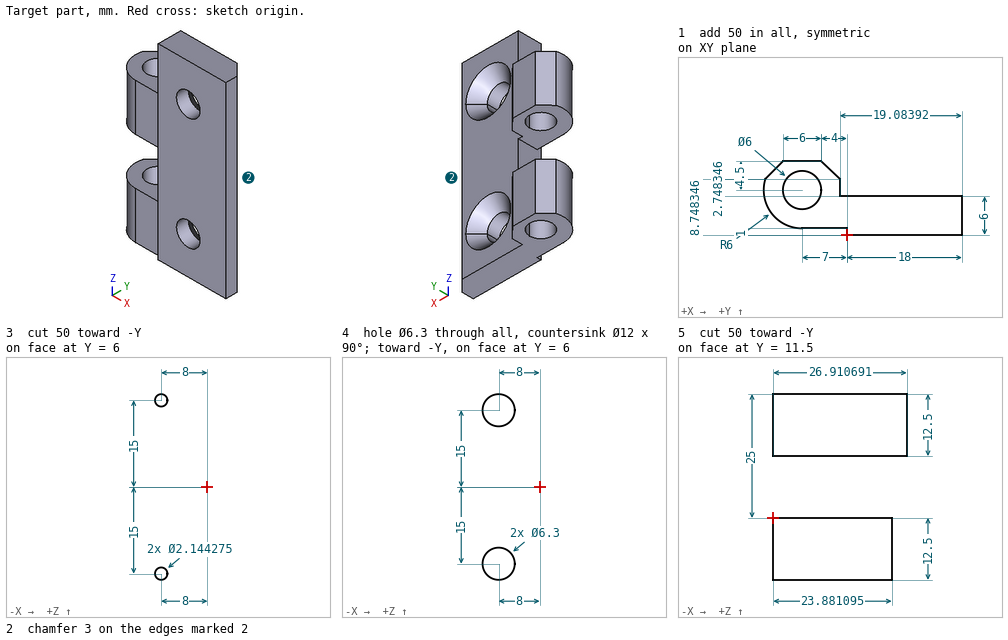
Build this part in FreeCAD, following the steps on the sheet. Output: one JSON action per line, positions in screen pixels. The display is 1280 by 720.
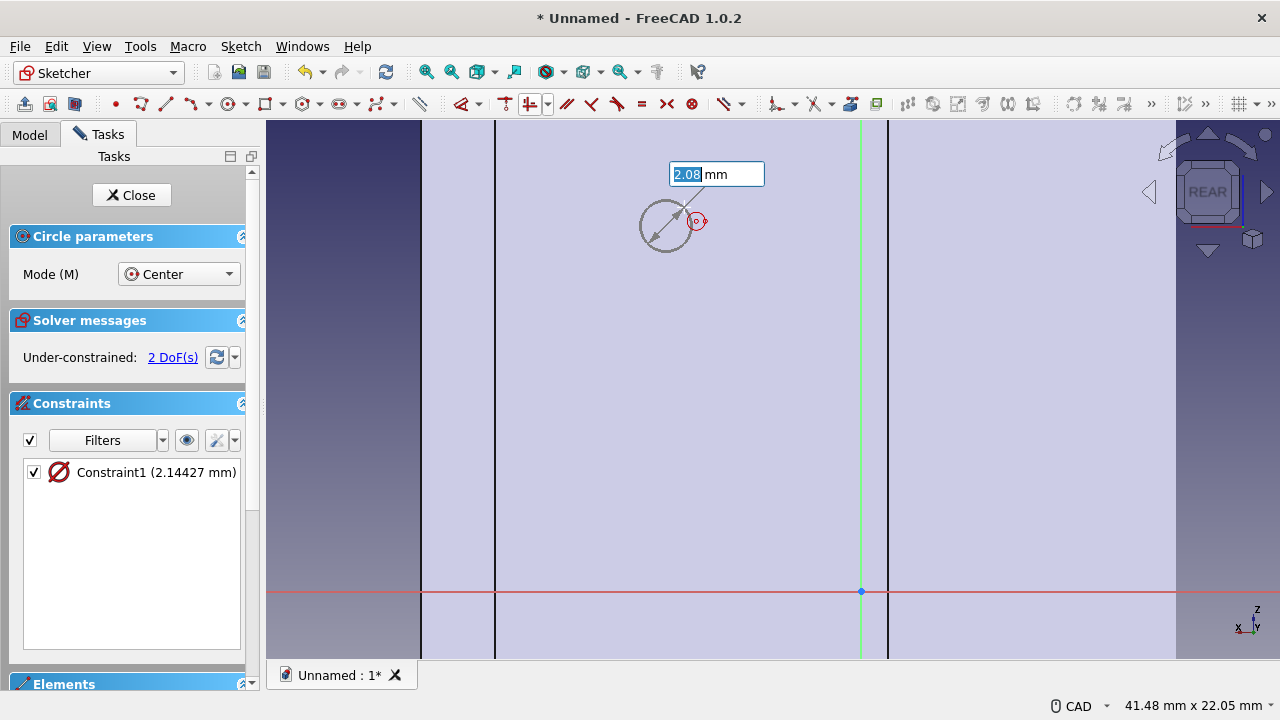
{"action": "type", "text": "2.144275"}
{"action": "key", "text": "Return"}
{"action": "key", "text": "Escape"}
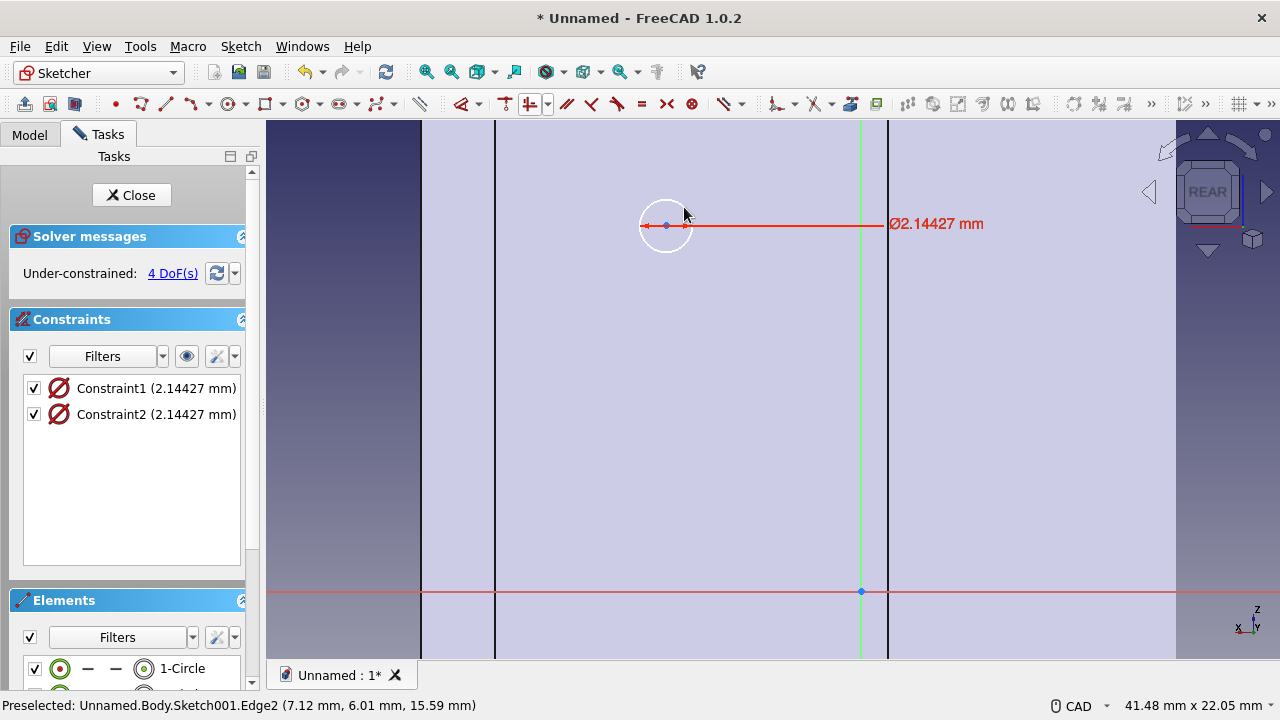
{"action": "left_click", "coordinate": [460, 104]}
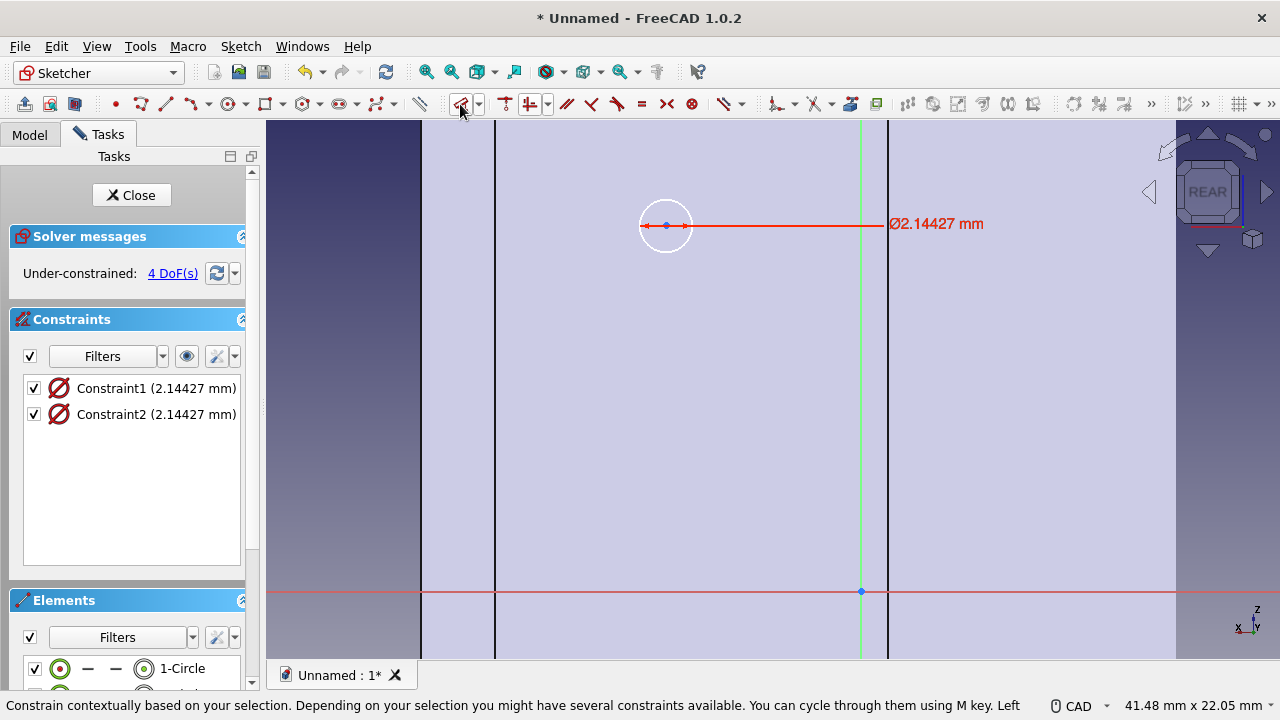
{"action": "scroll", "coordinate": [667, 224], "scroll_direction": "down", "scroll_amount": 4}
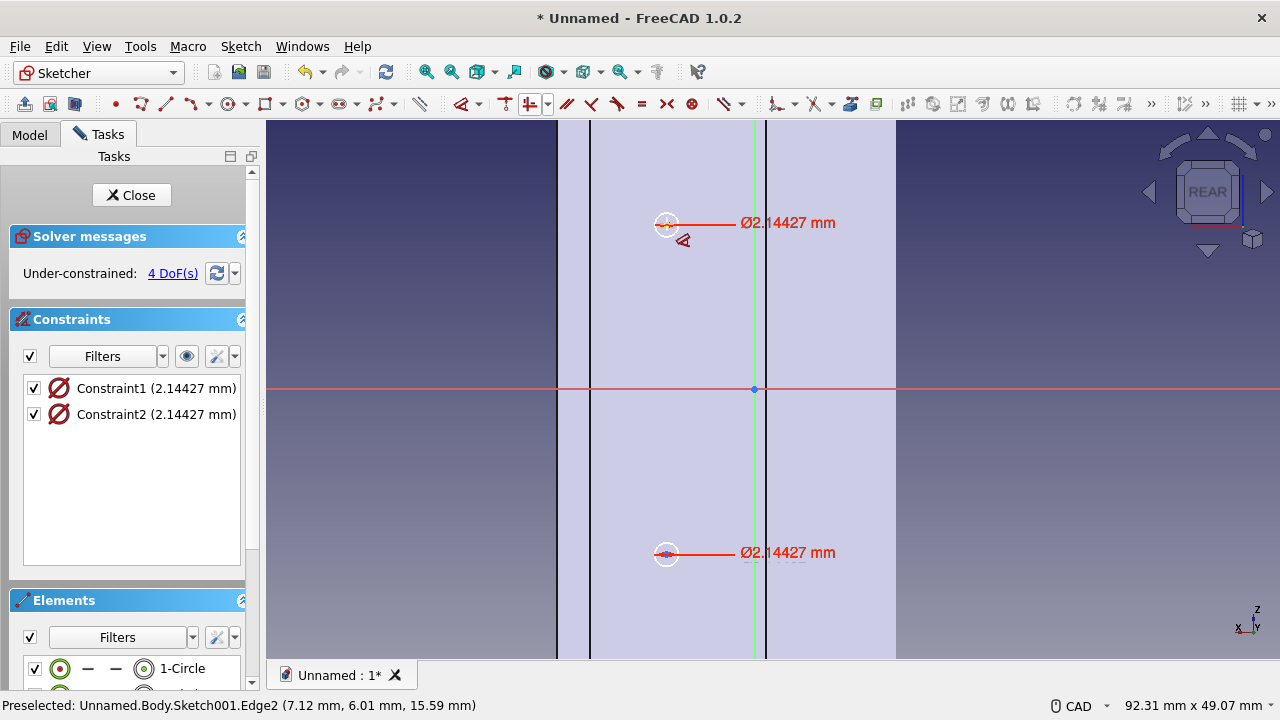
{"action": "left_click", "coordinate": [667, 555]}
{"action": "left_click", "coordinate": [711, 589]}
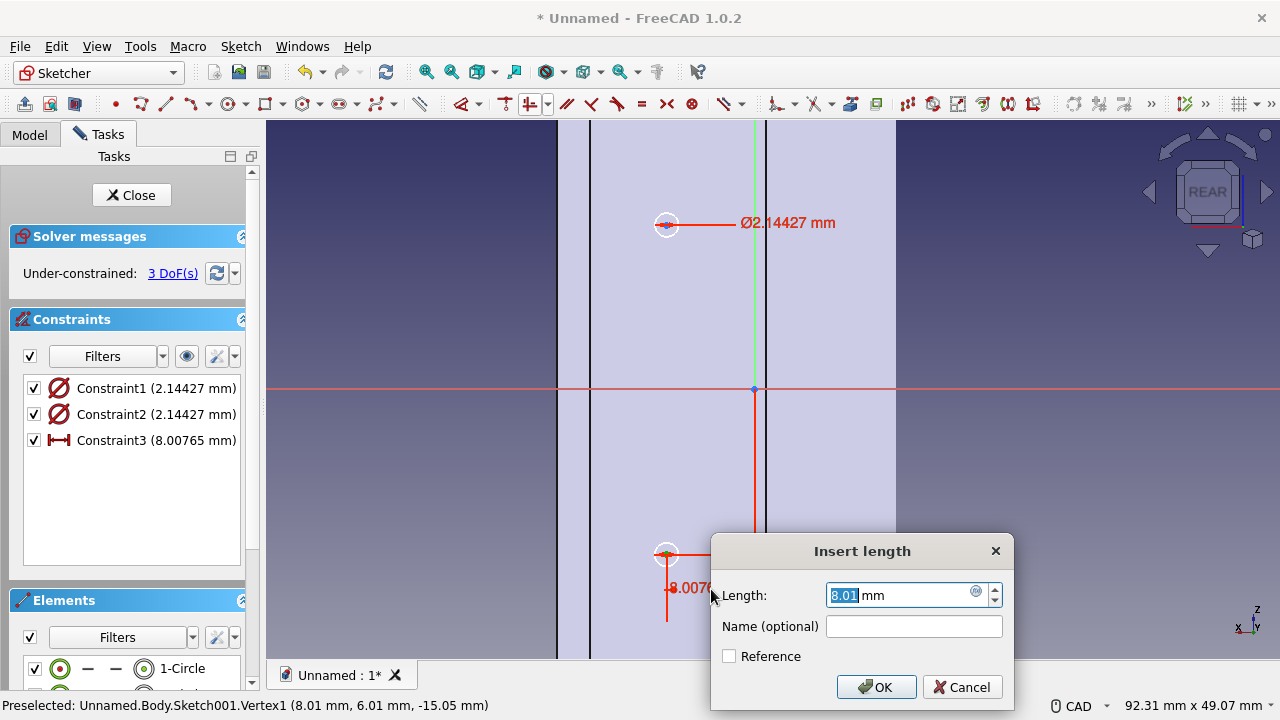
{"action": "type", "text": "8"}
{"action": "key", "text": "Return"}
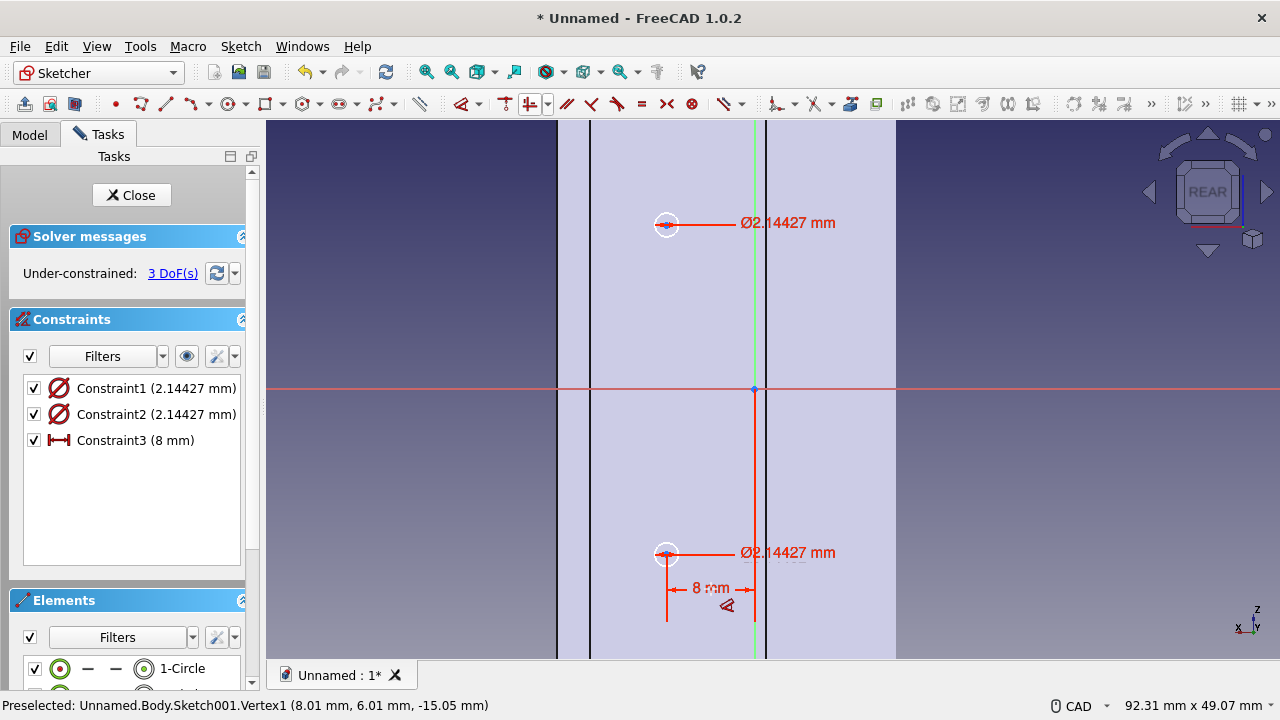
{"action": "left_click", "coordinate": [667, 225]}
{"action": "left_click", "coordinate": [711, 191]}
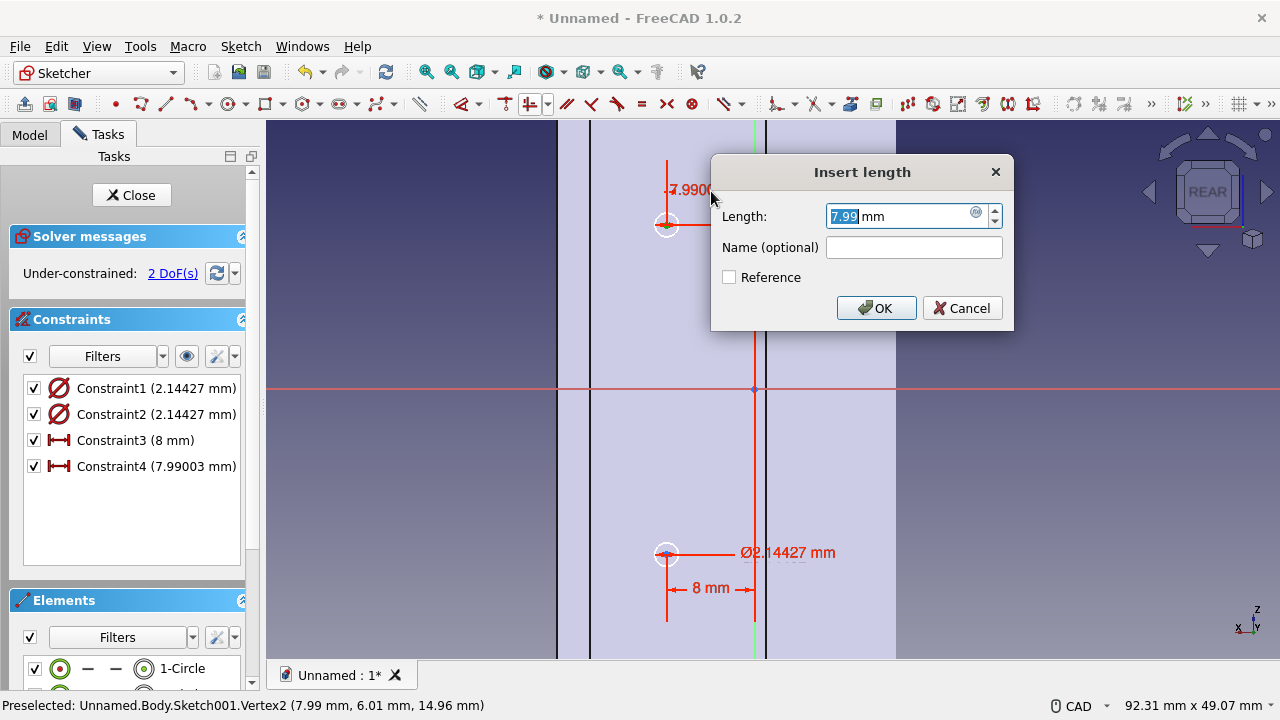
{"action": "type", "text": "8"}
{"action": "key", "text": "Return"}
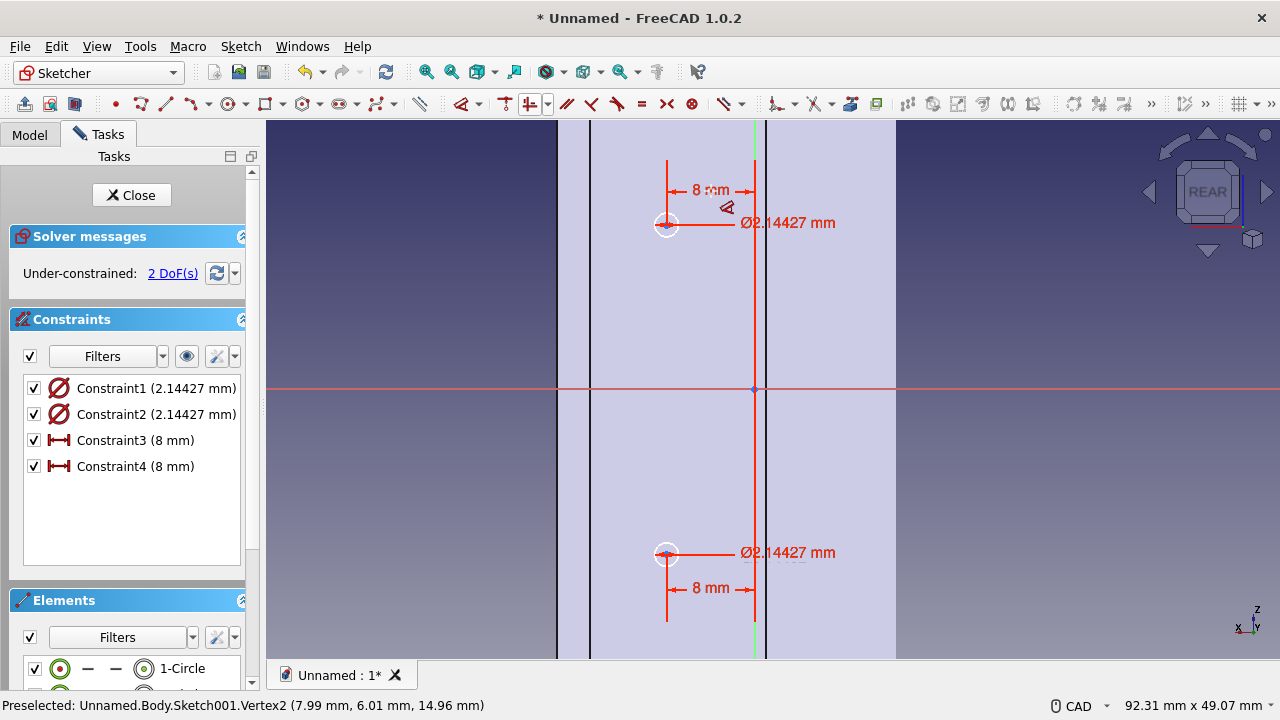
{"action": "left_click", "coordinate": [667, 555]}
{"action": "left_click", "coordinate": [789, 472]}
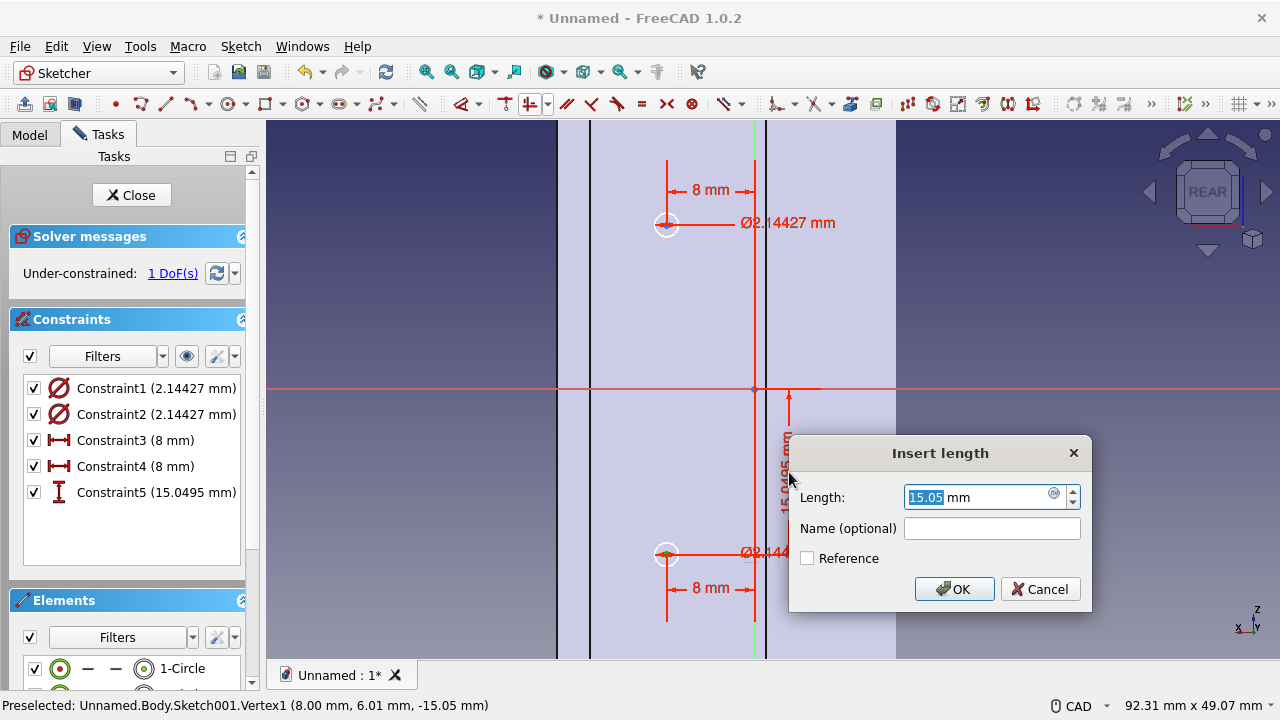
{"action": "type", "text": "15"}
{"action": "key", "text": "Return"}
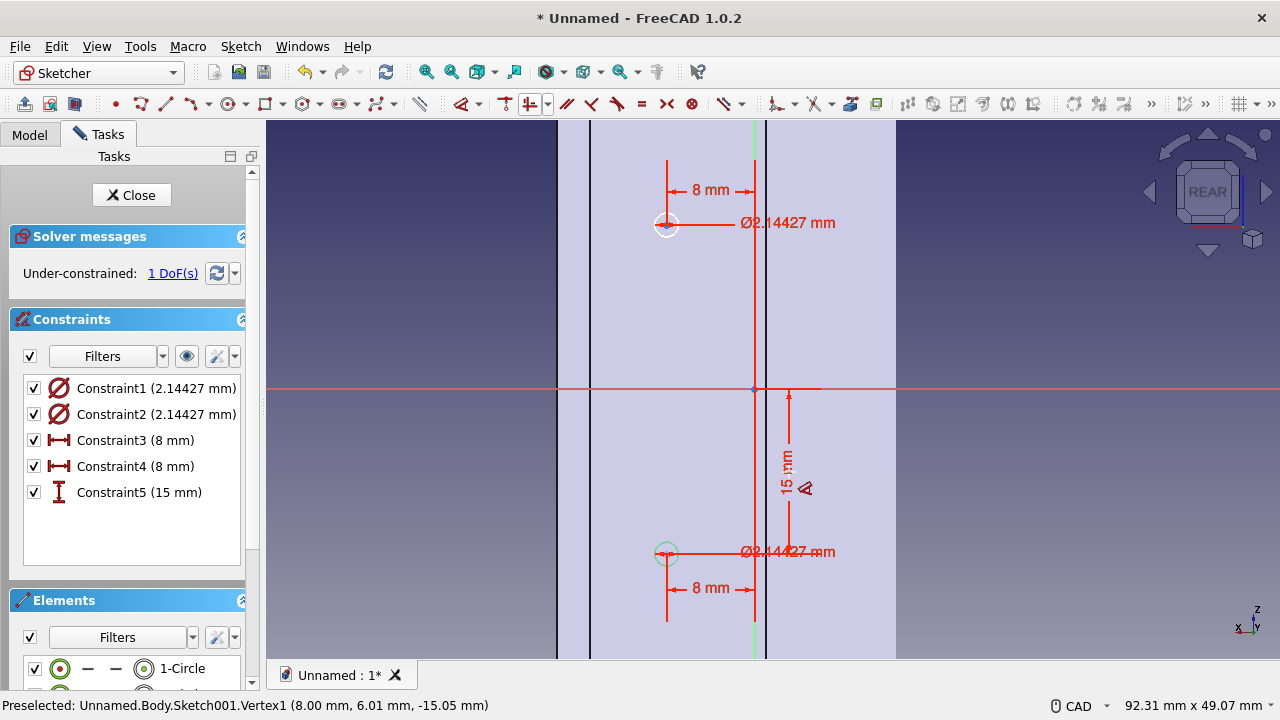
{"action": "left_click", "coordinate": [667, 225]}
{"action": "left_click", "coordinate": [789, 307]}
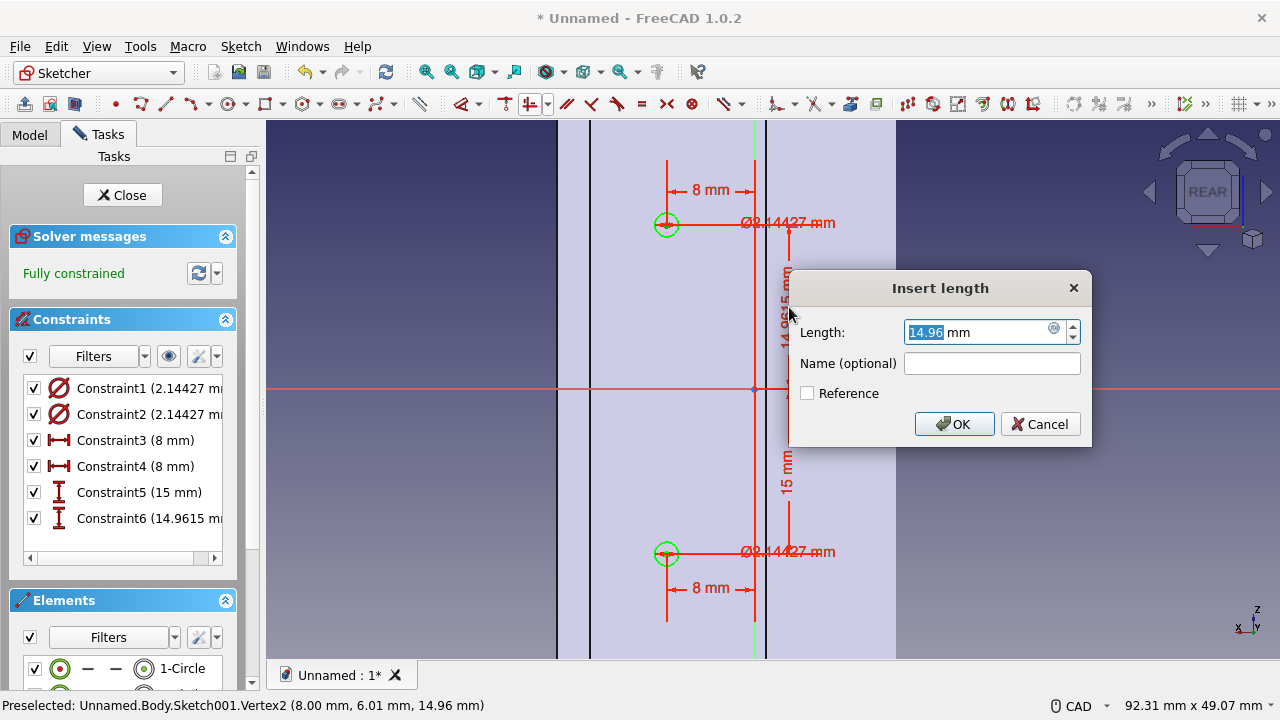
{"action": "type", "text": "15"}
{"action": "key", "text": "Return"}
{"action": "key", "text": "Escape"}